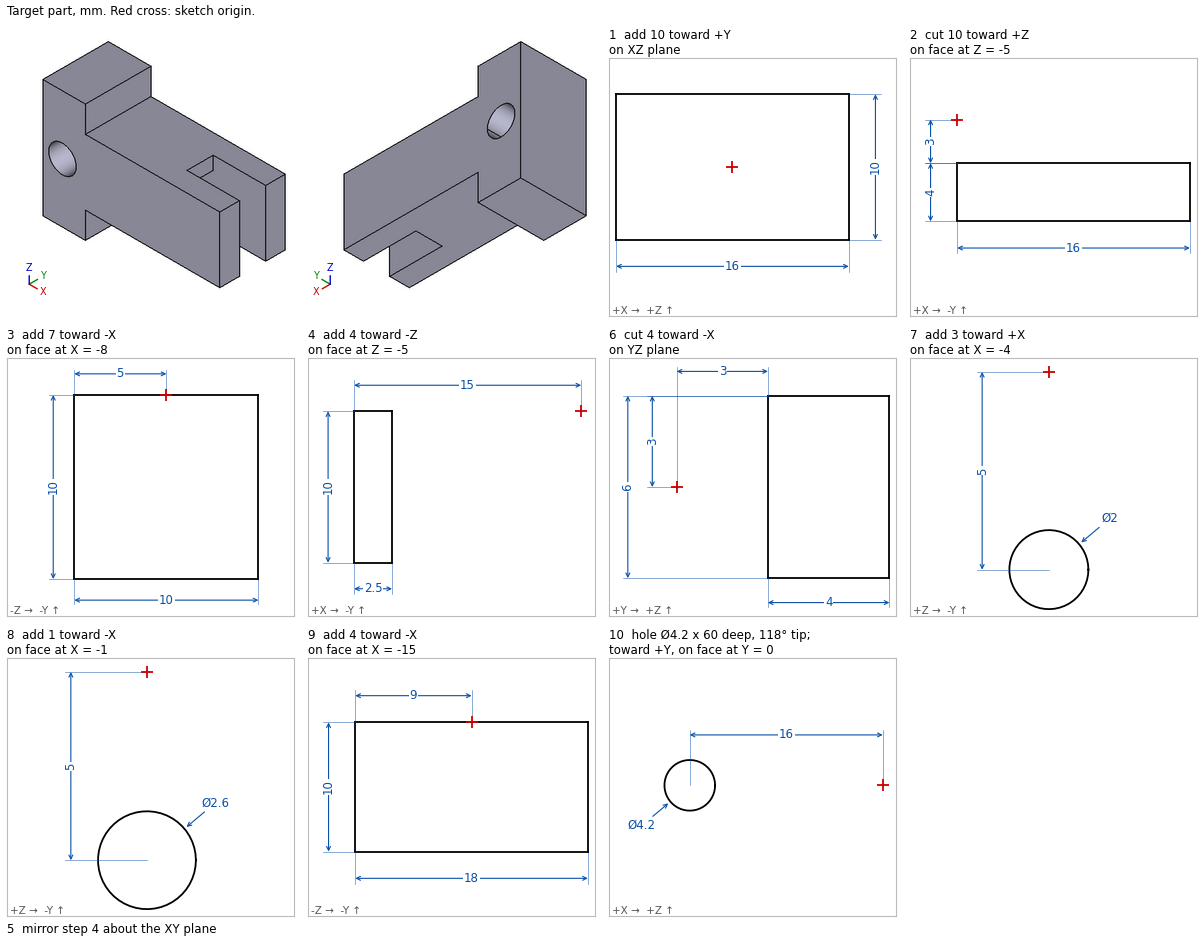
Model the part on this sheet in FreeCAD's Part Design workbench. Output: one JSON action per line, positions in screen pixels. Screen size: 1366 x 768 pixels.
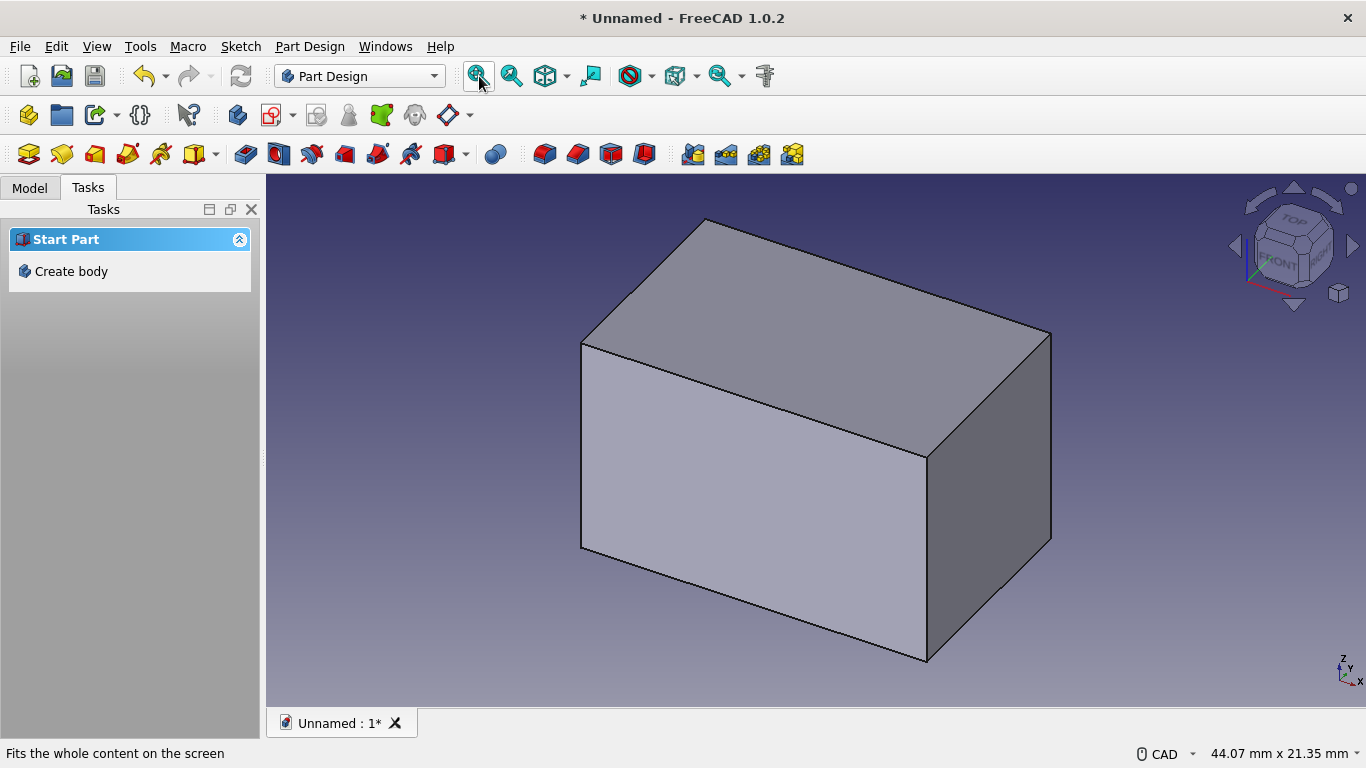
{"action": "key", "text": "5"}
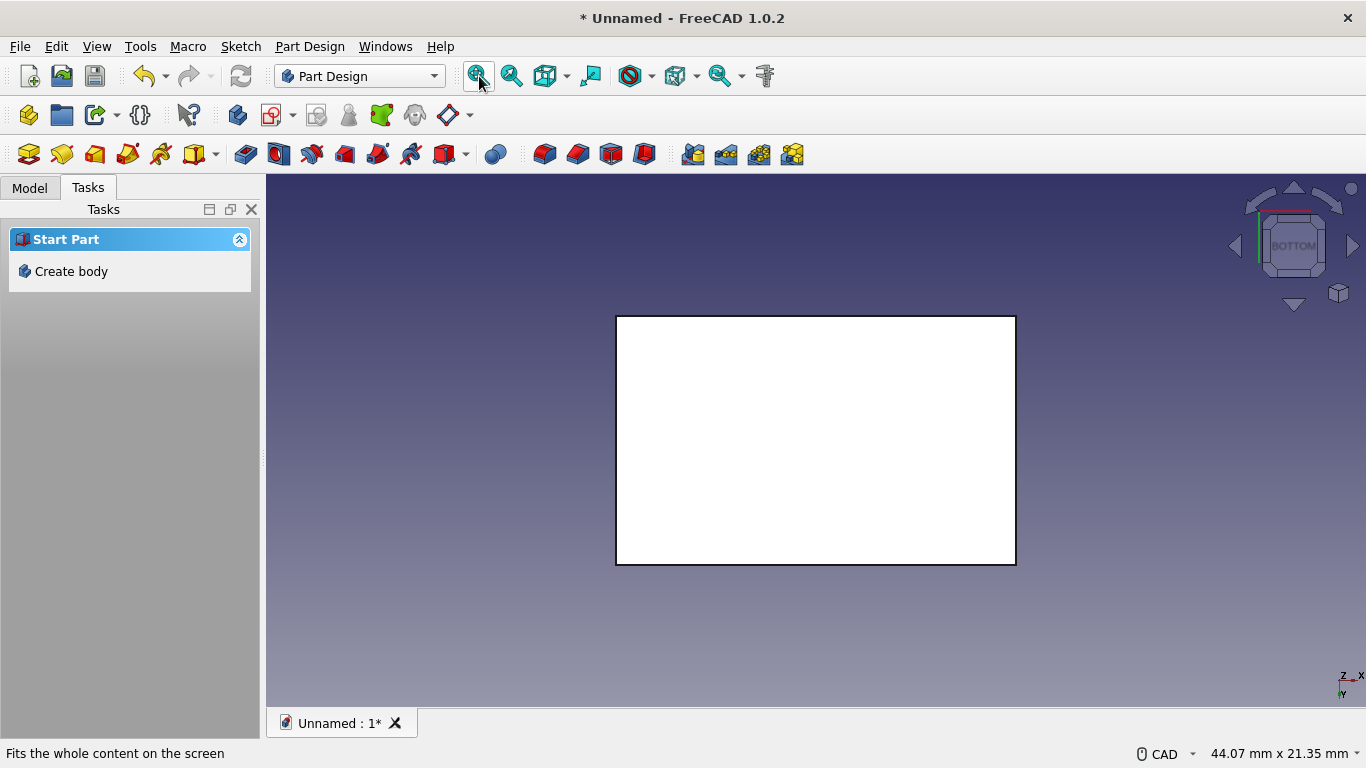
{"action": "left_click", "coordinate": [873, 439]}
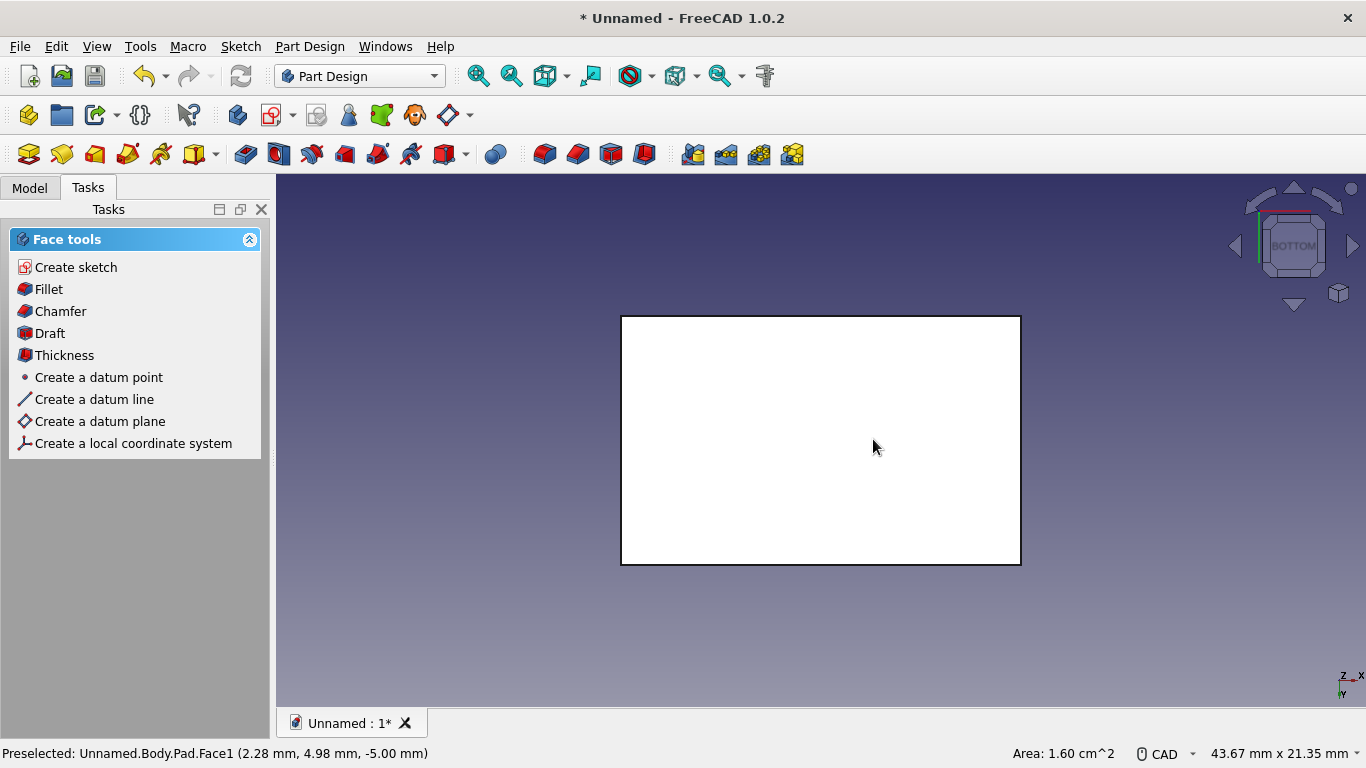
{"action": "left_click", "coordinate": [270, 116]}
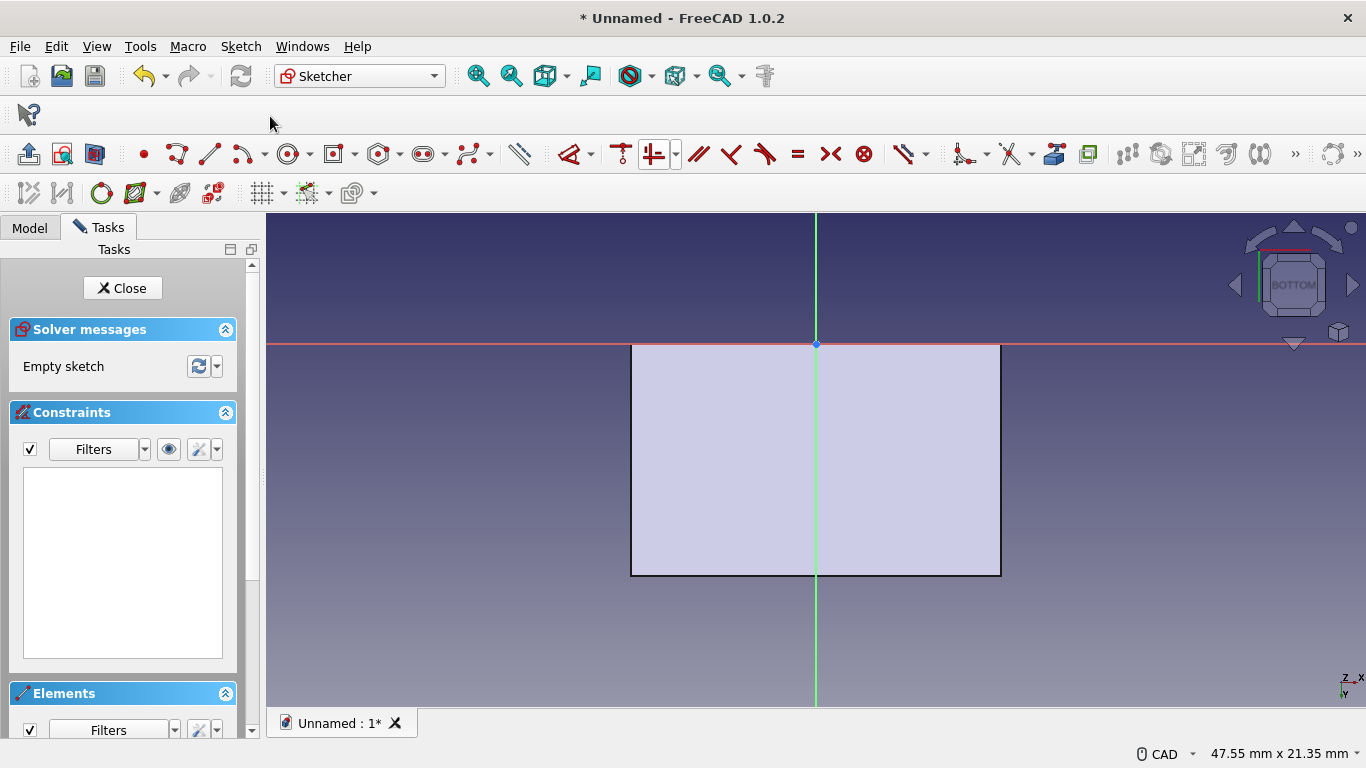
{"action": "scroll", "coordinate": [1201, 383], "scroll_direction": "up", "scroll_amount": 3}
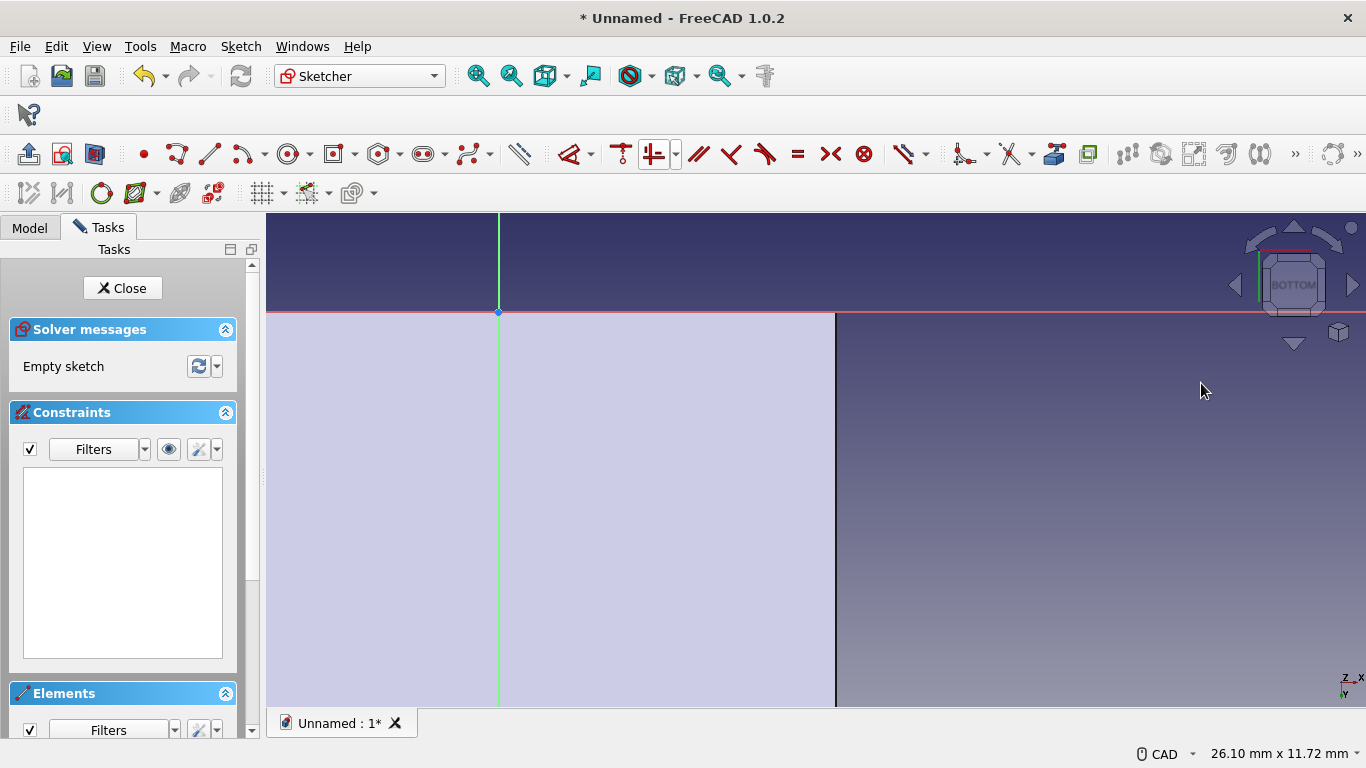
{"action": "left_click", "coordinate": [354, 154]}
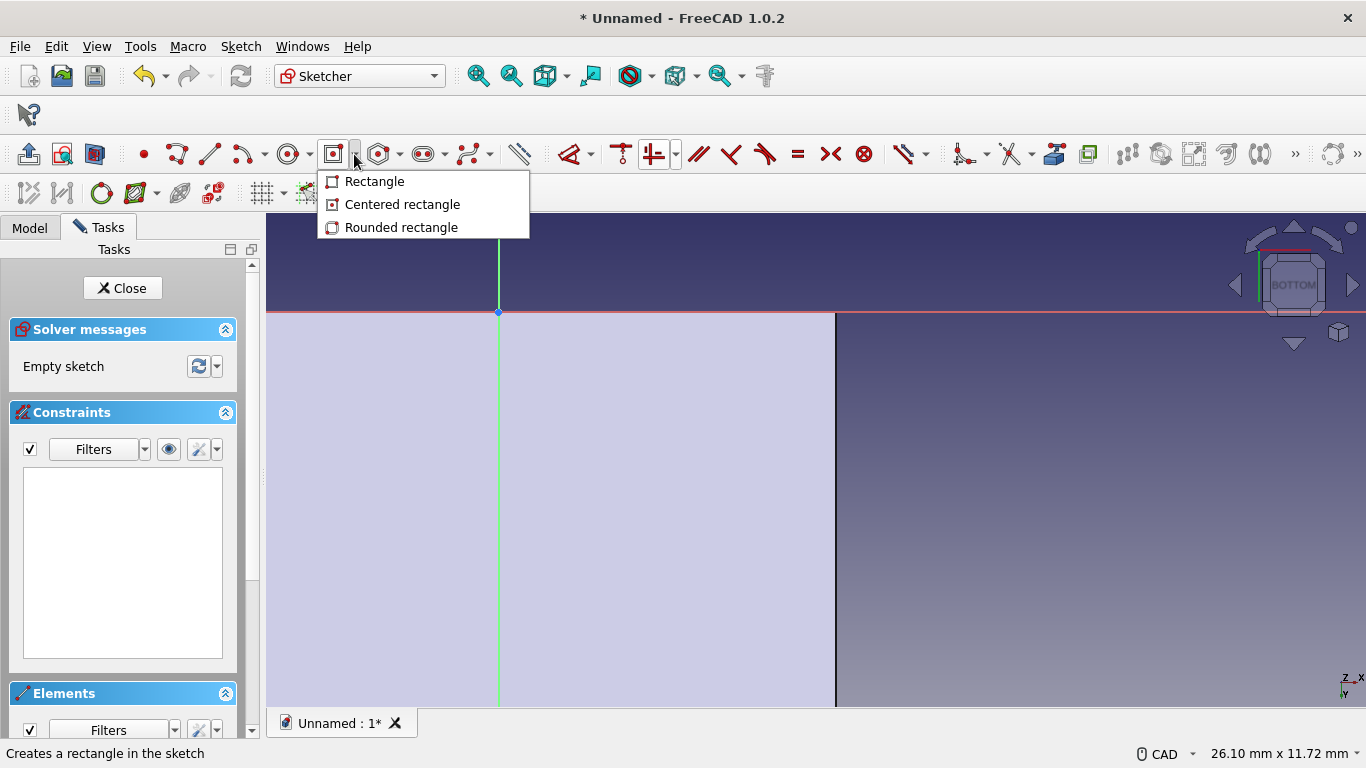
{"action": "left_click", "coordinate": [424, 182]}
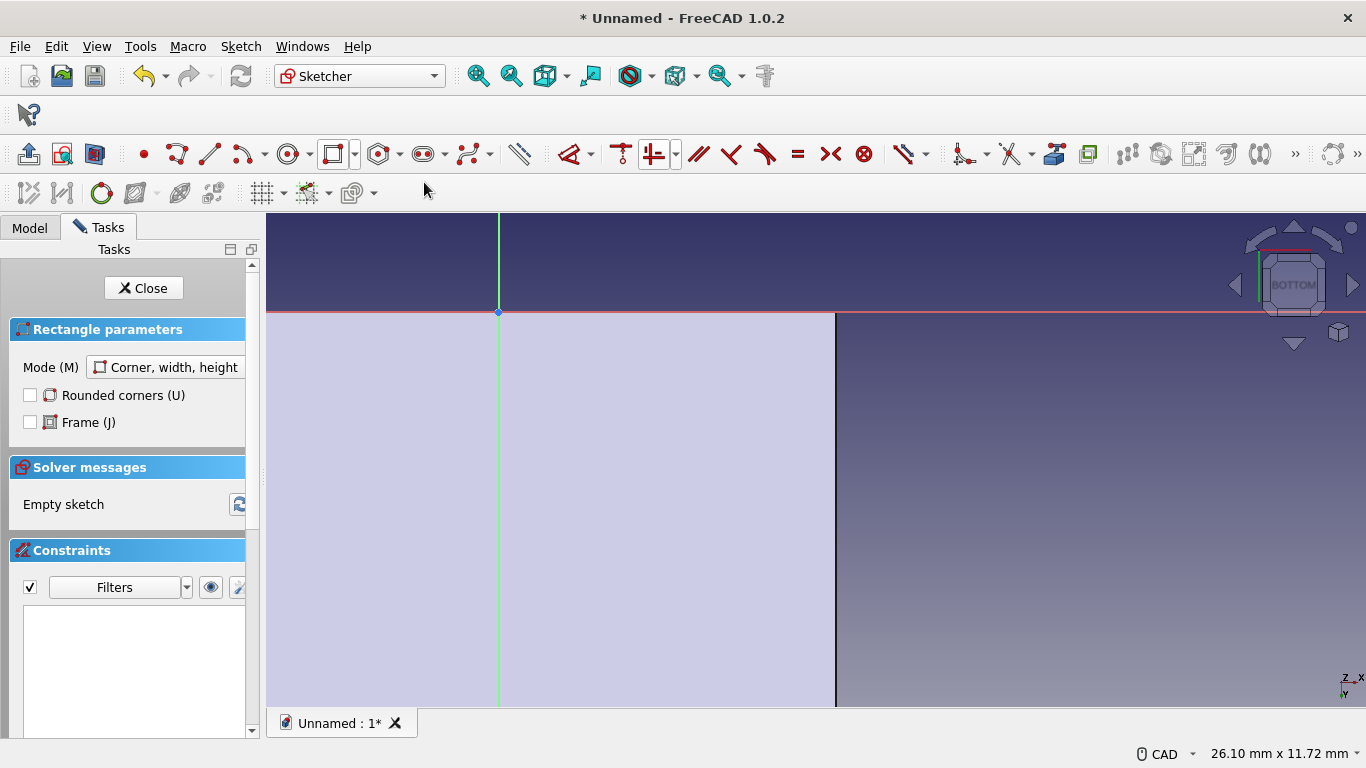
{"action": "left_click", "coordinate": [499, 439]}
{"action": "left_click", "coordinate": [1173, 607]}
{"action": "key", "text": "Escape"}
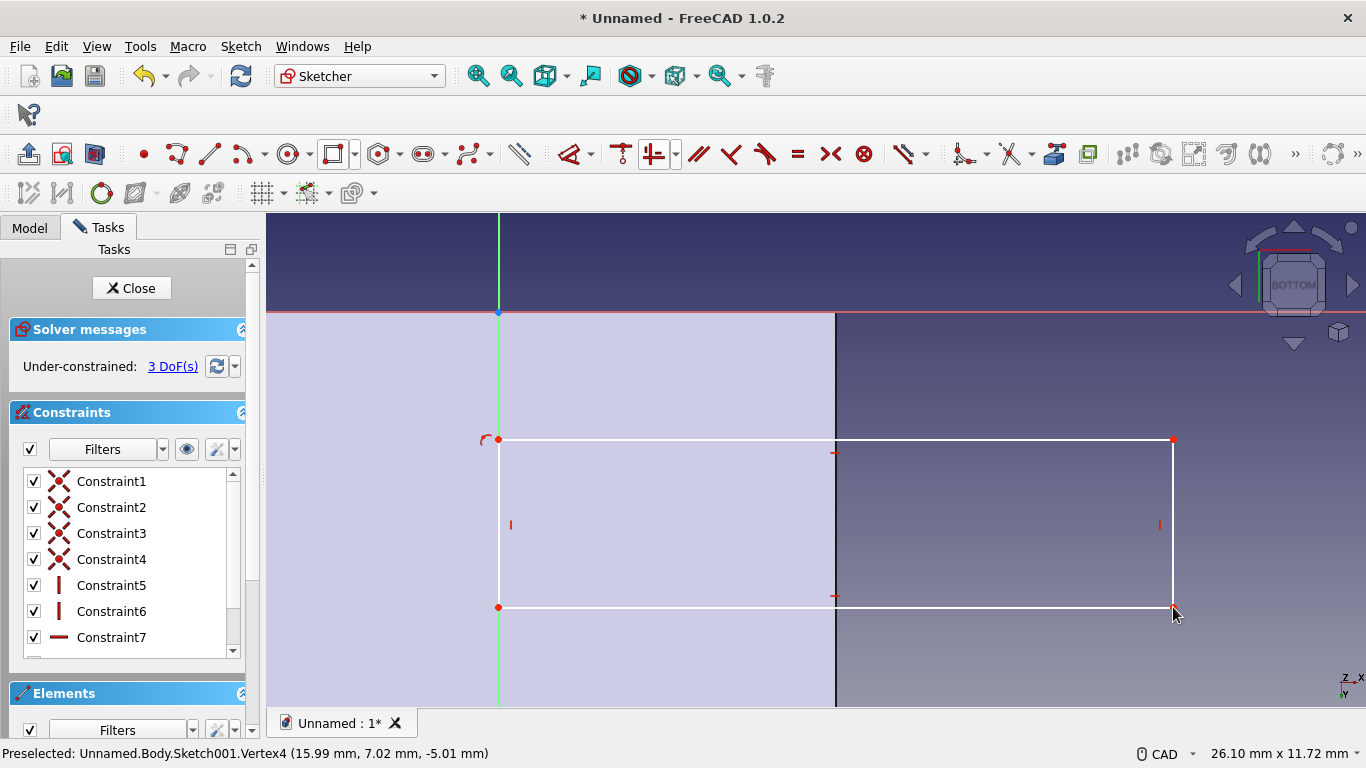
{"action": "left_click", "coordinate": [568, 154]}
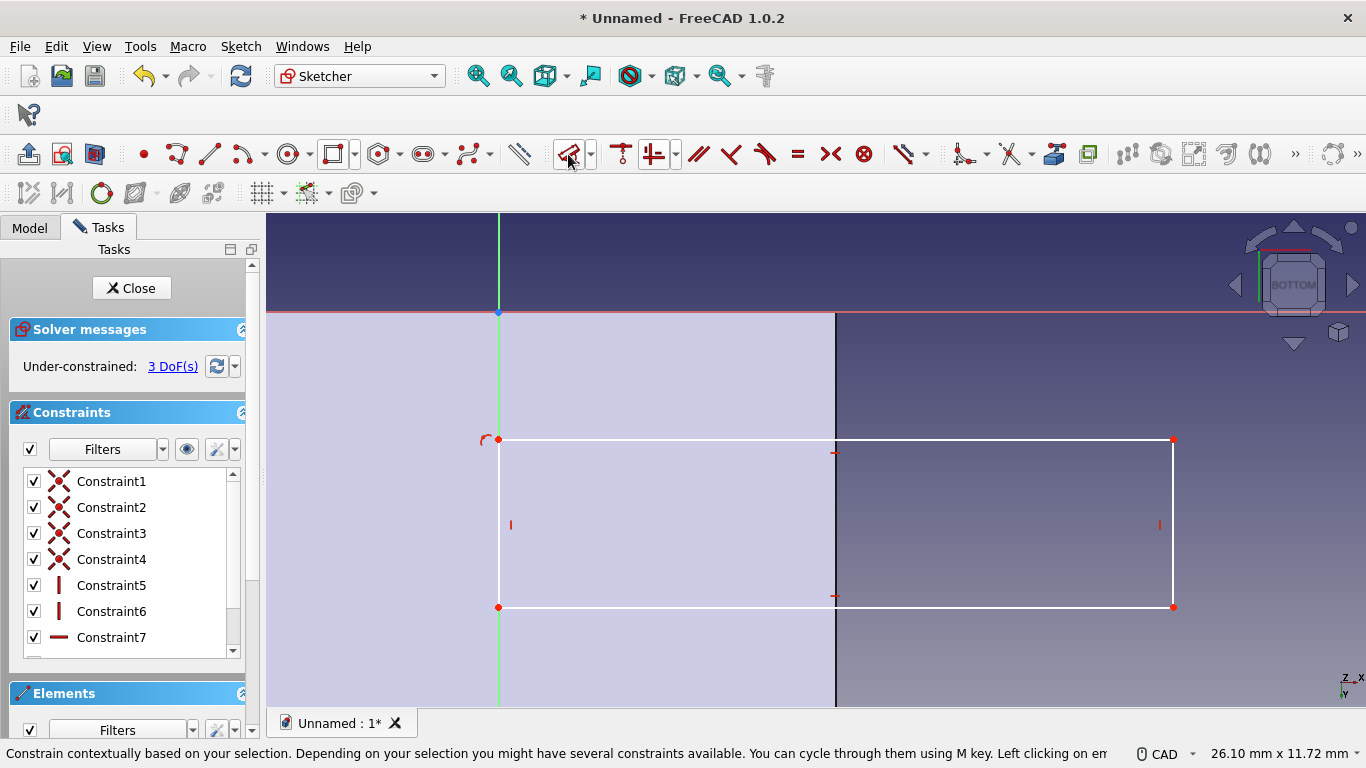
{"action": "left_click", "coordinate": [499, 490]}
{"action": "left_click", "coordinate": [465, 524]}